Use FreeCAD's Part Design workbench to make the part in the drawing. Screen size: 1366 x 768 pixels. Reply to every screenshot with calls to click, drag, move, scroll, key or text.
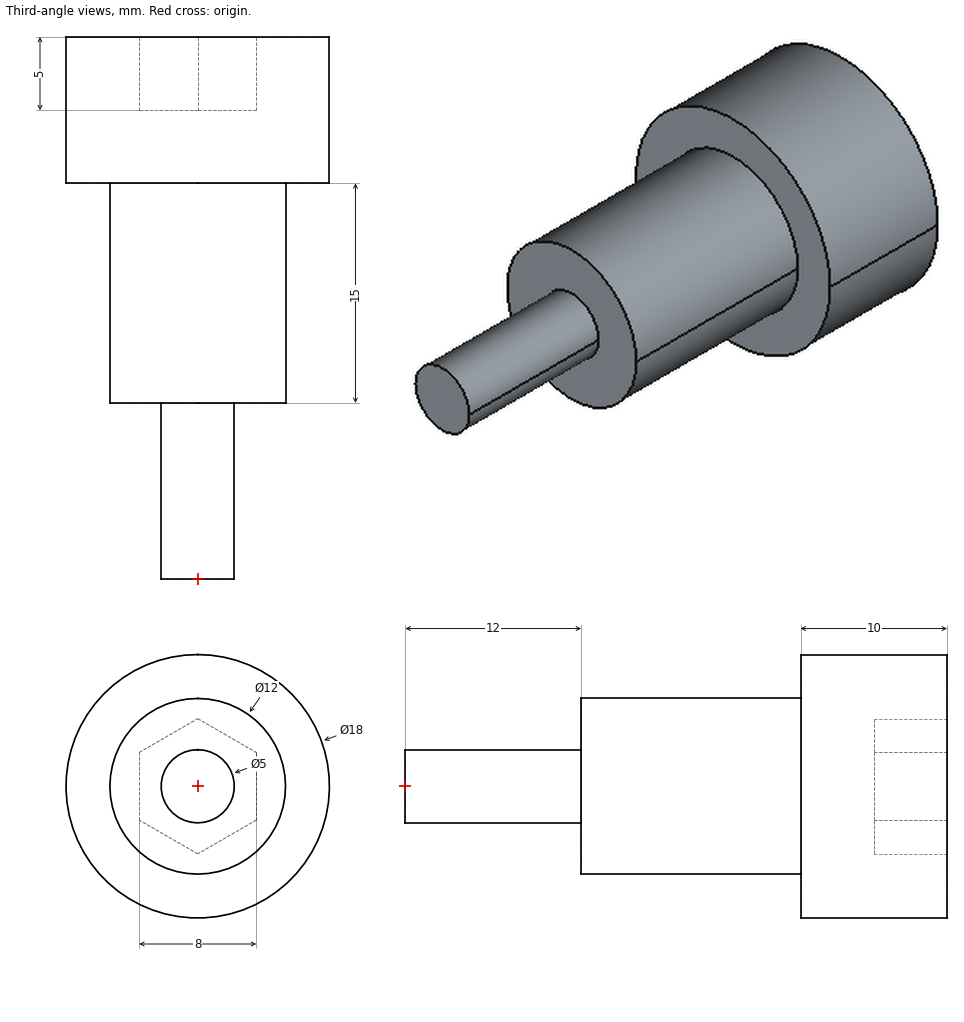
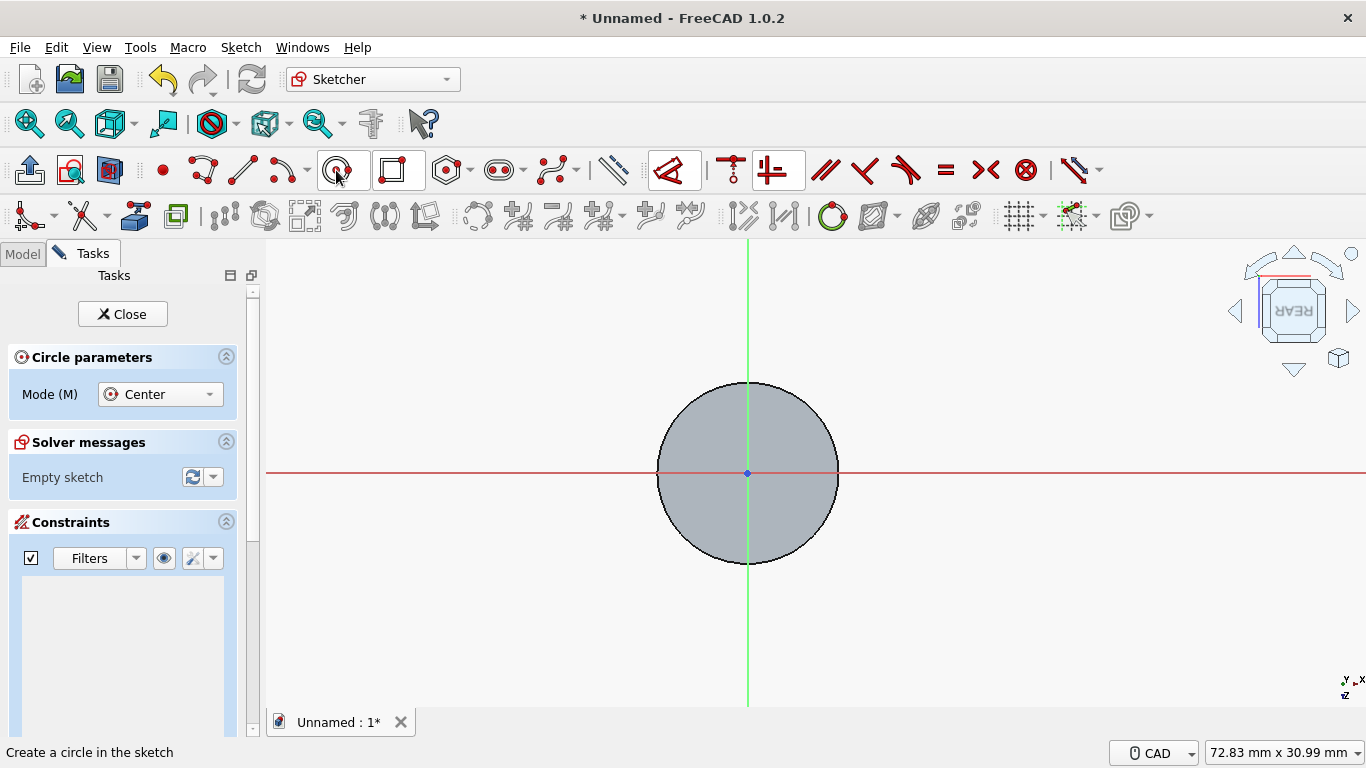
click(748, 473)
move(844, 377)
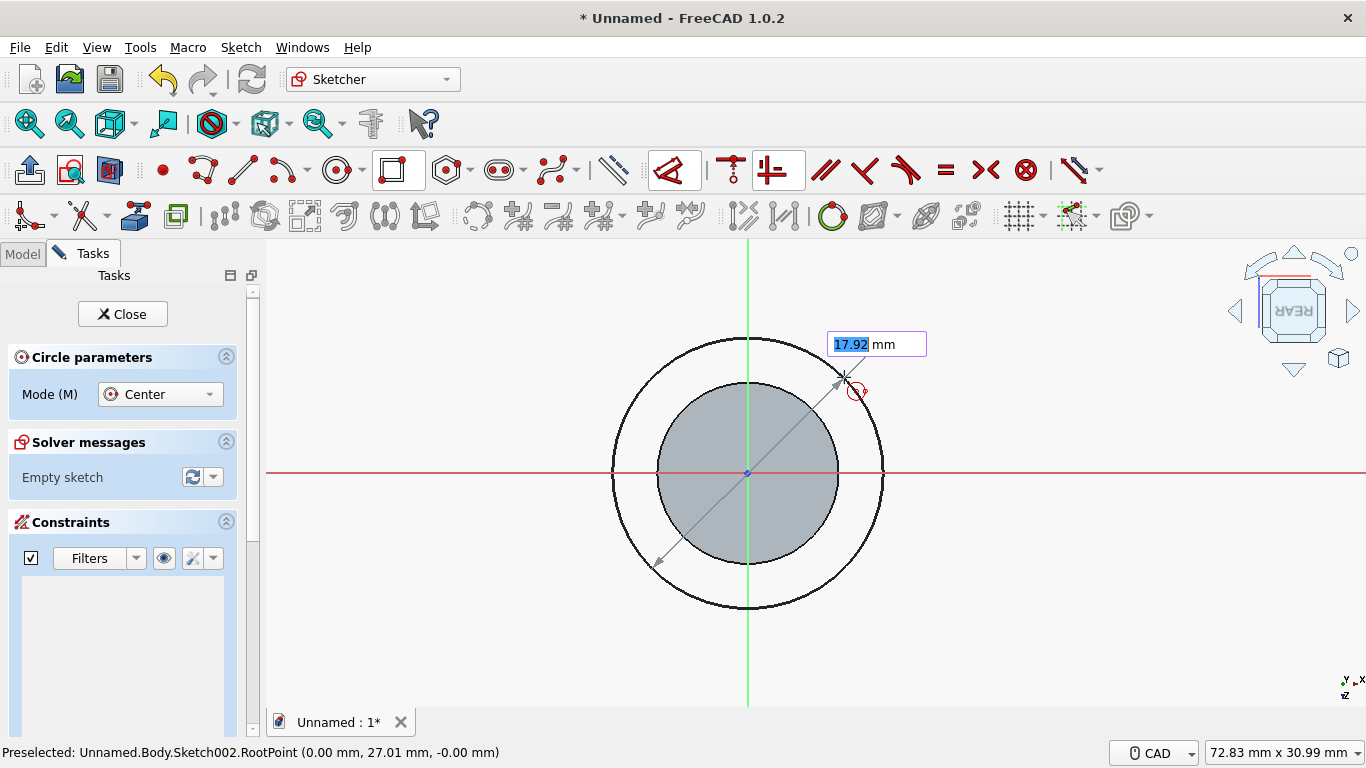
text(18)
key(Return)
key(Escape)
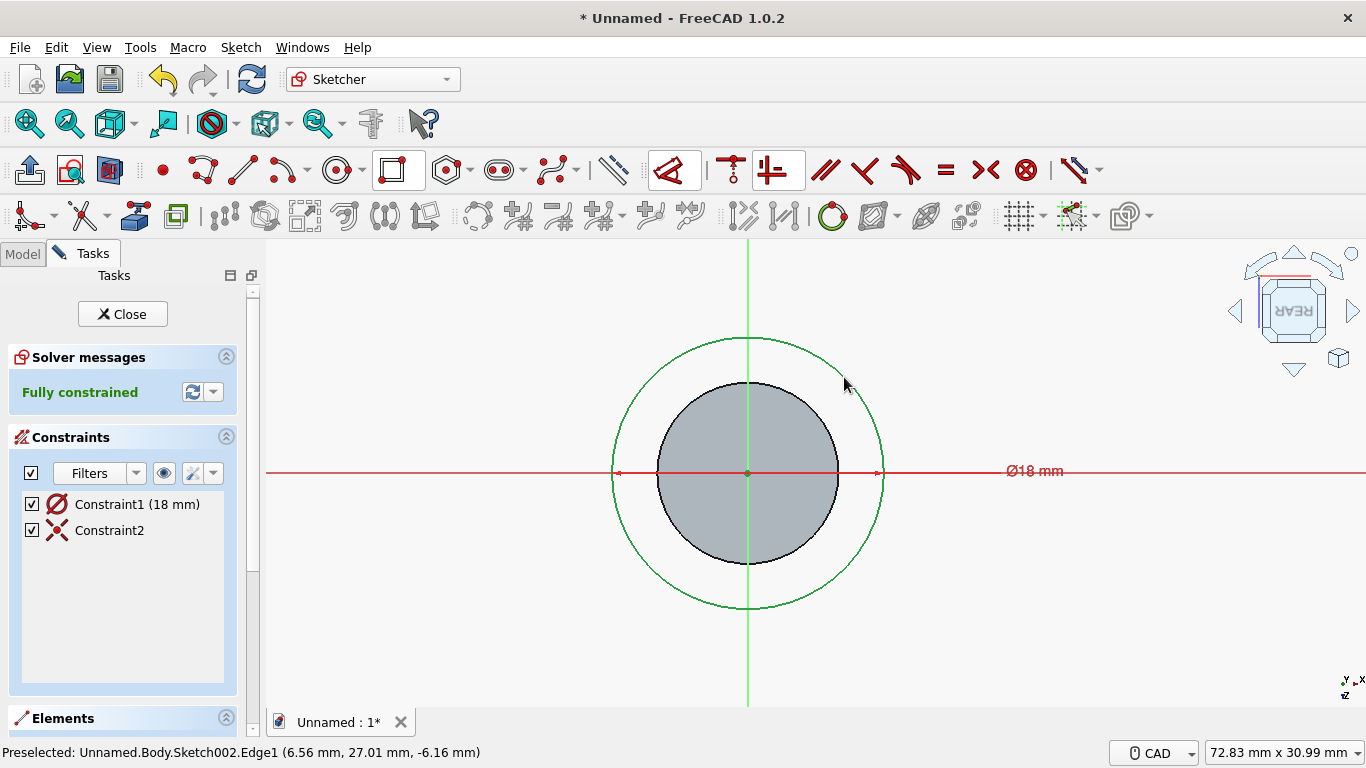
click(123, 314)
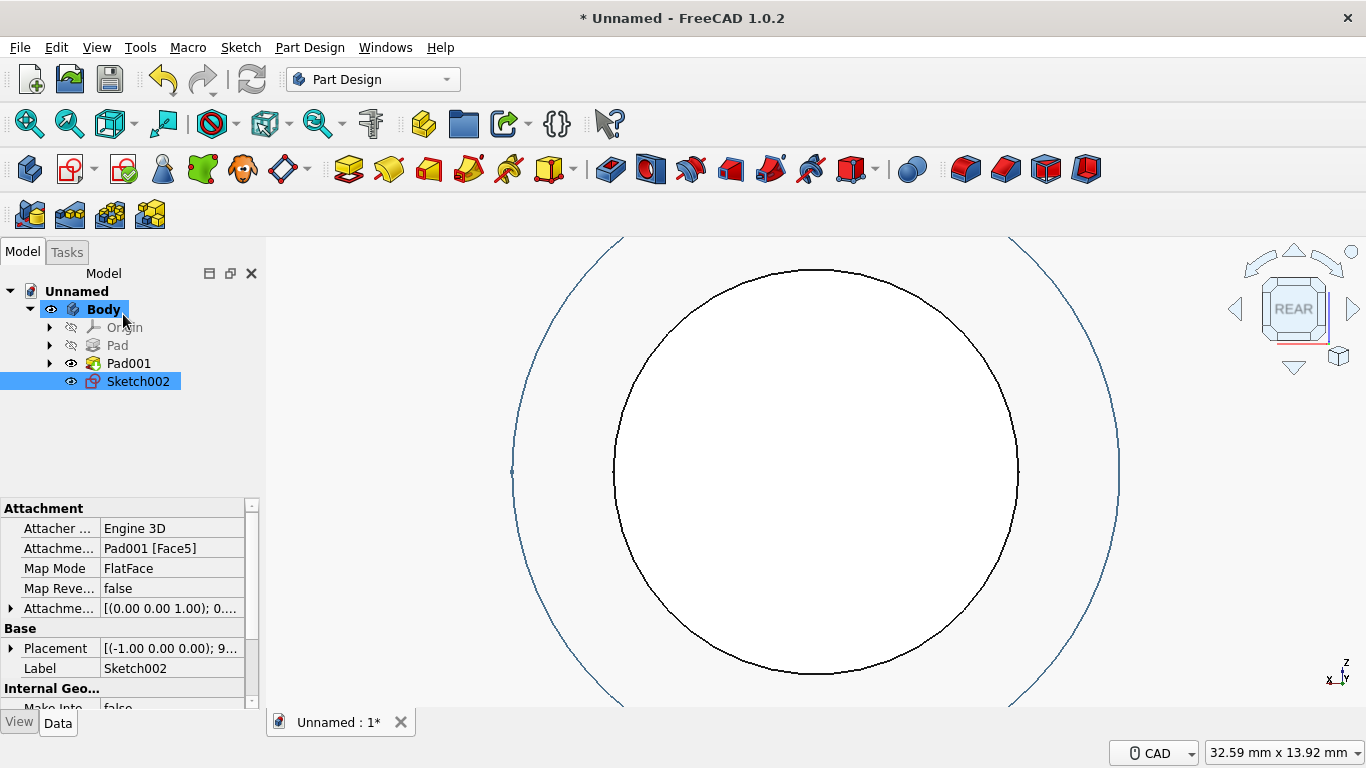
click(350, 170)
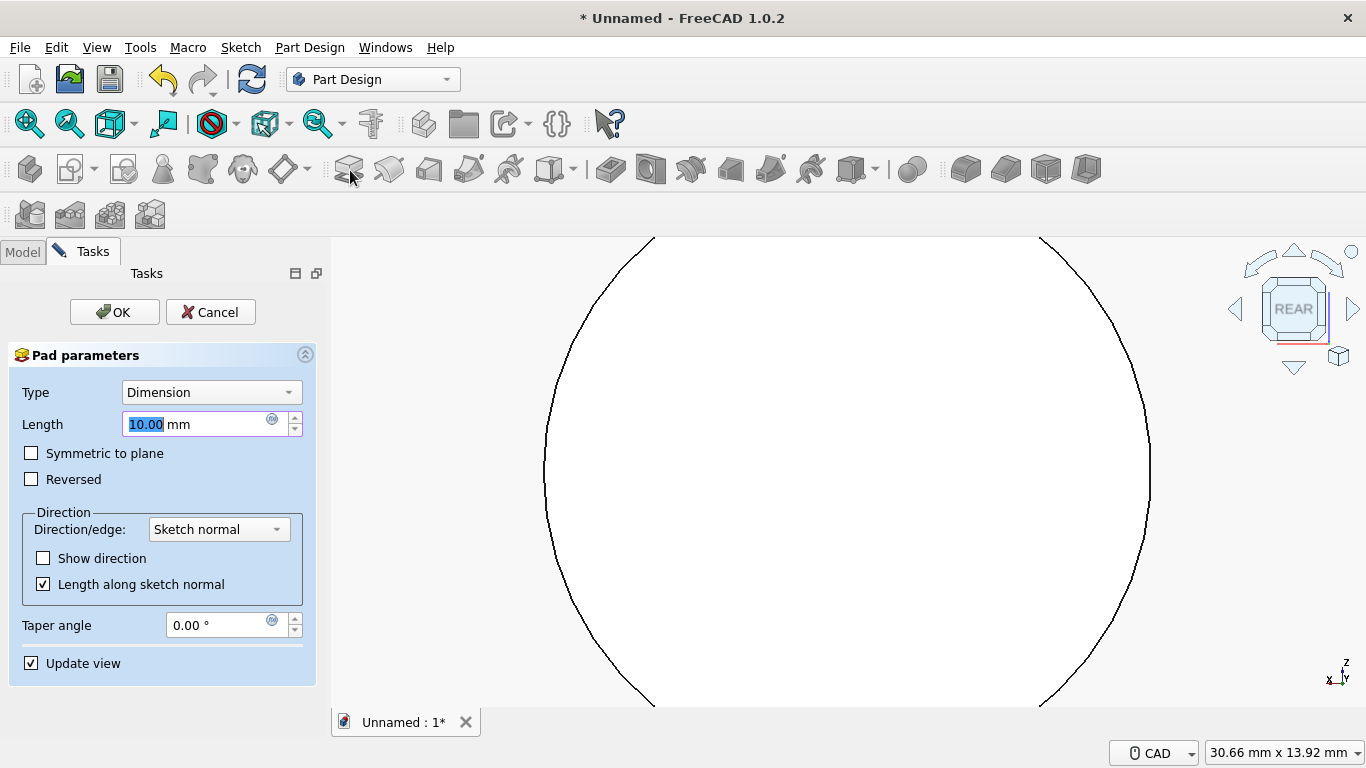
text(10)
key(Tab)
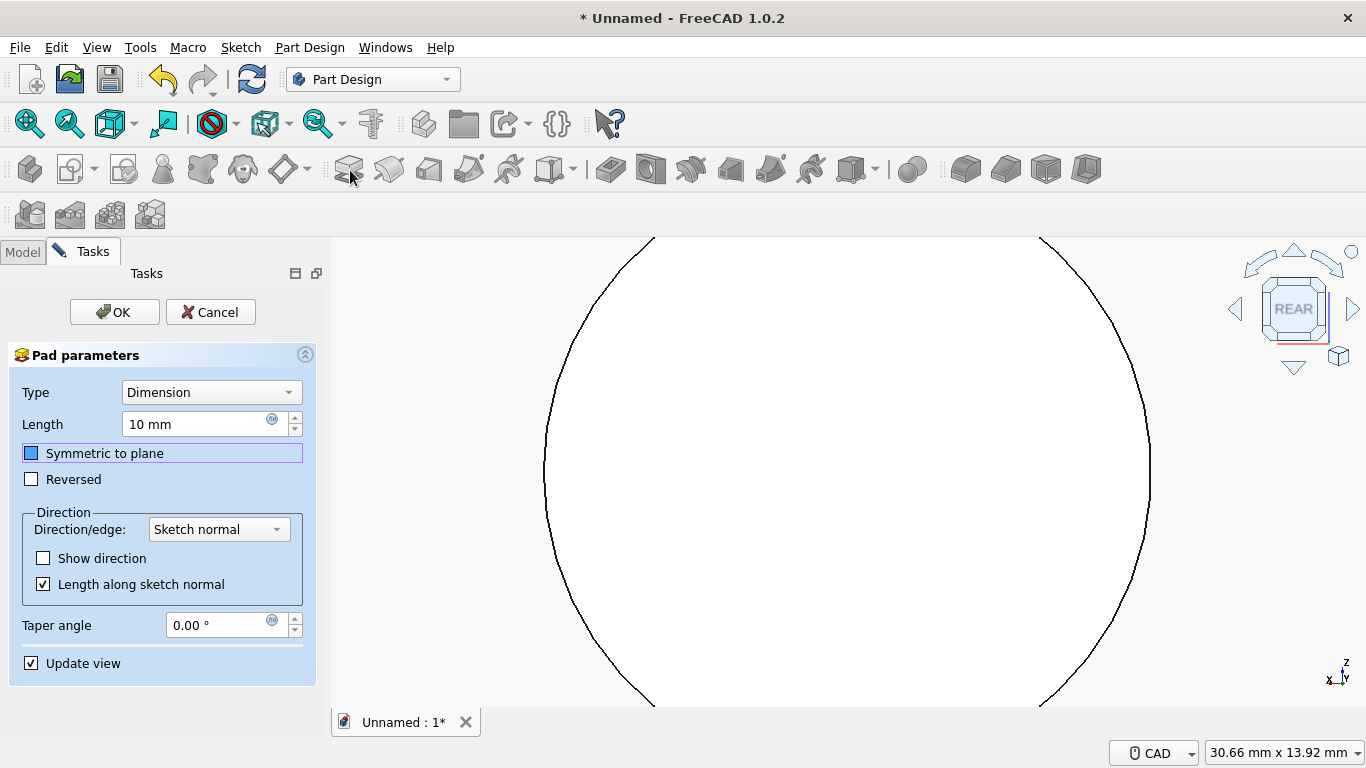
click(115, 312)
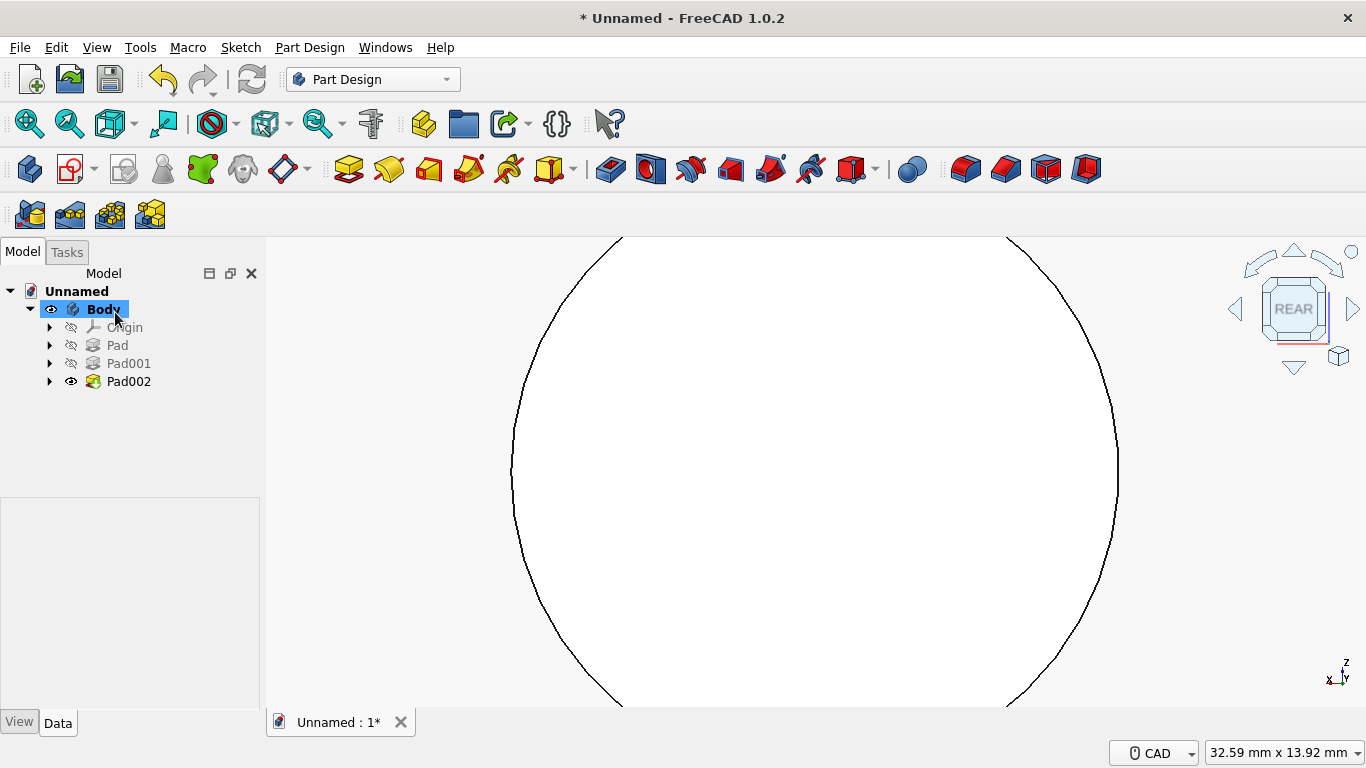
click(30, 124)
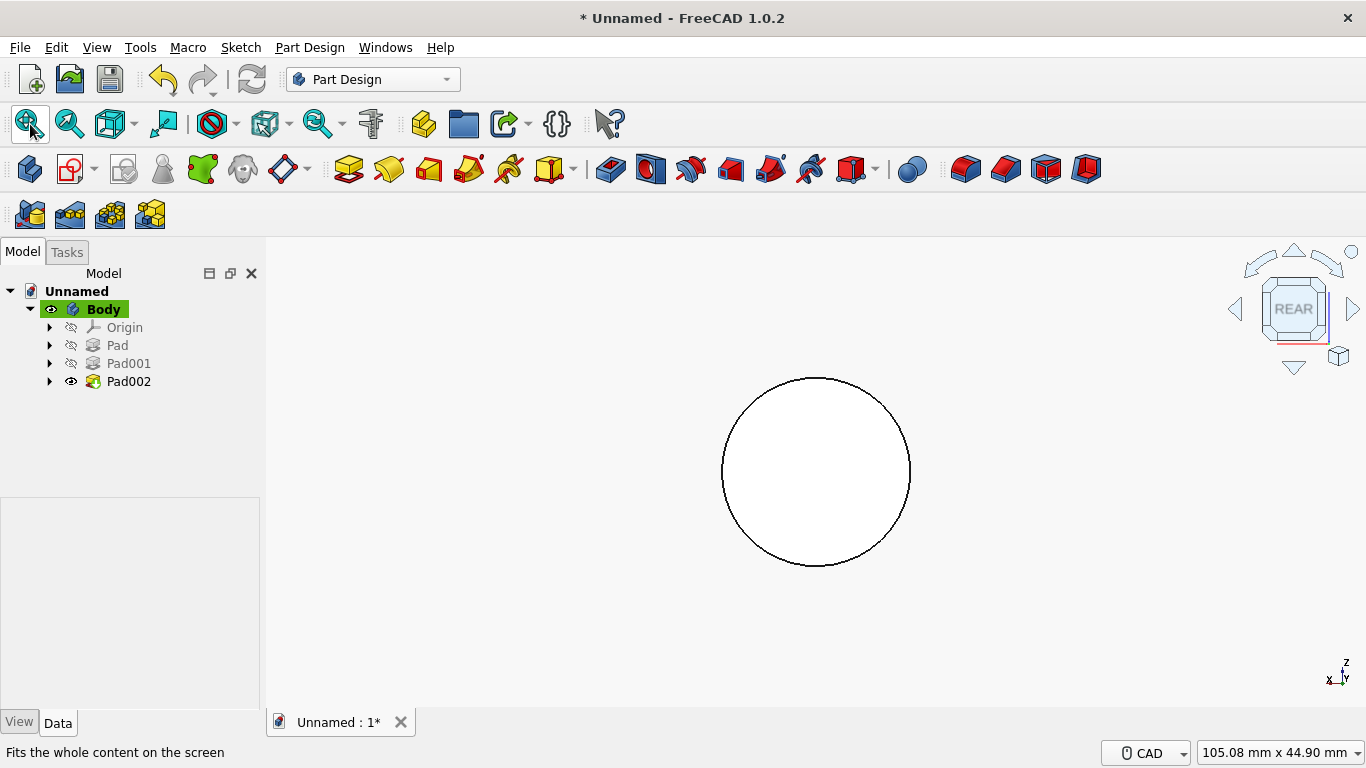
click(816, 471)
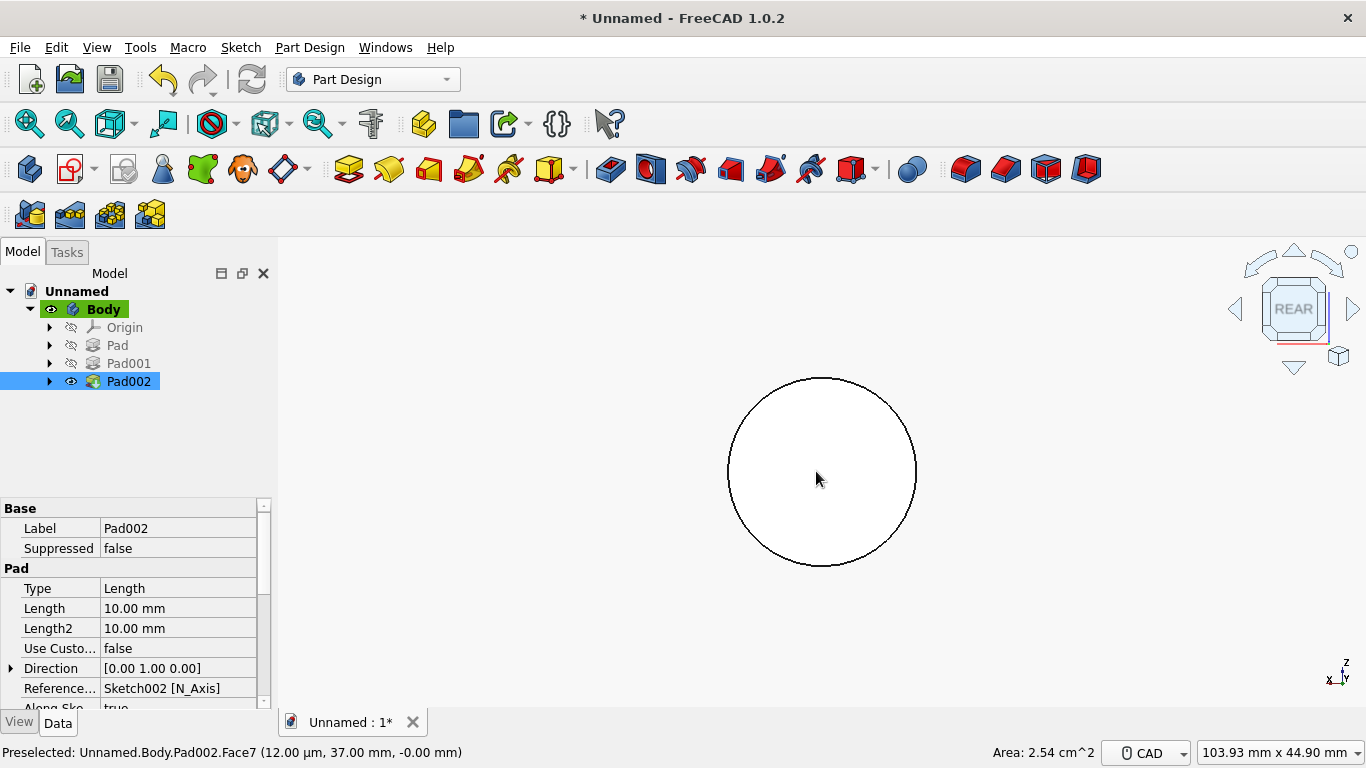
click(70, 170)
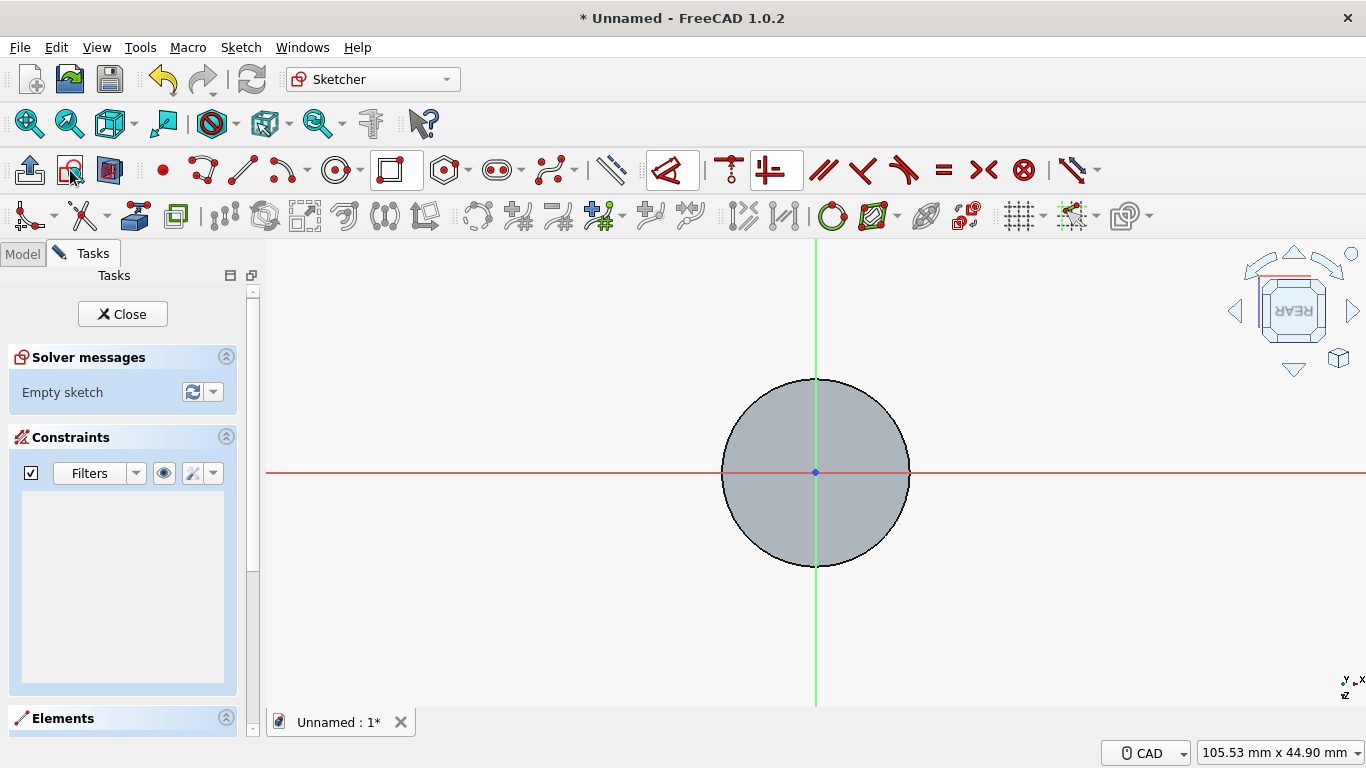
scroll(845, 473, up, 6)